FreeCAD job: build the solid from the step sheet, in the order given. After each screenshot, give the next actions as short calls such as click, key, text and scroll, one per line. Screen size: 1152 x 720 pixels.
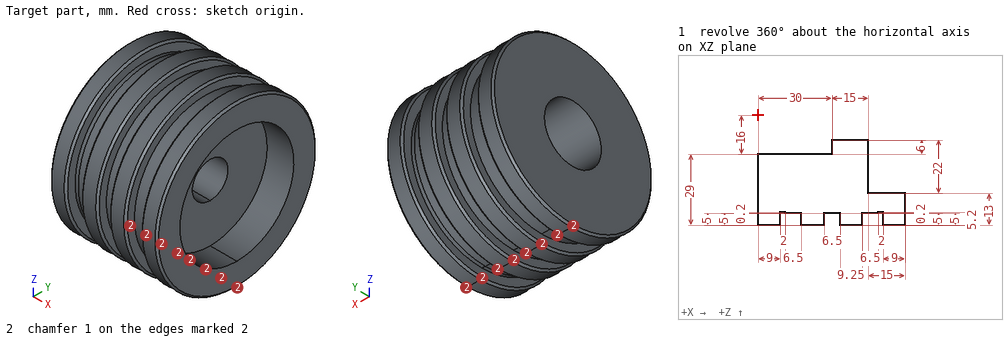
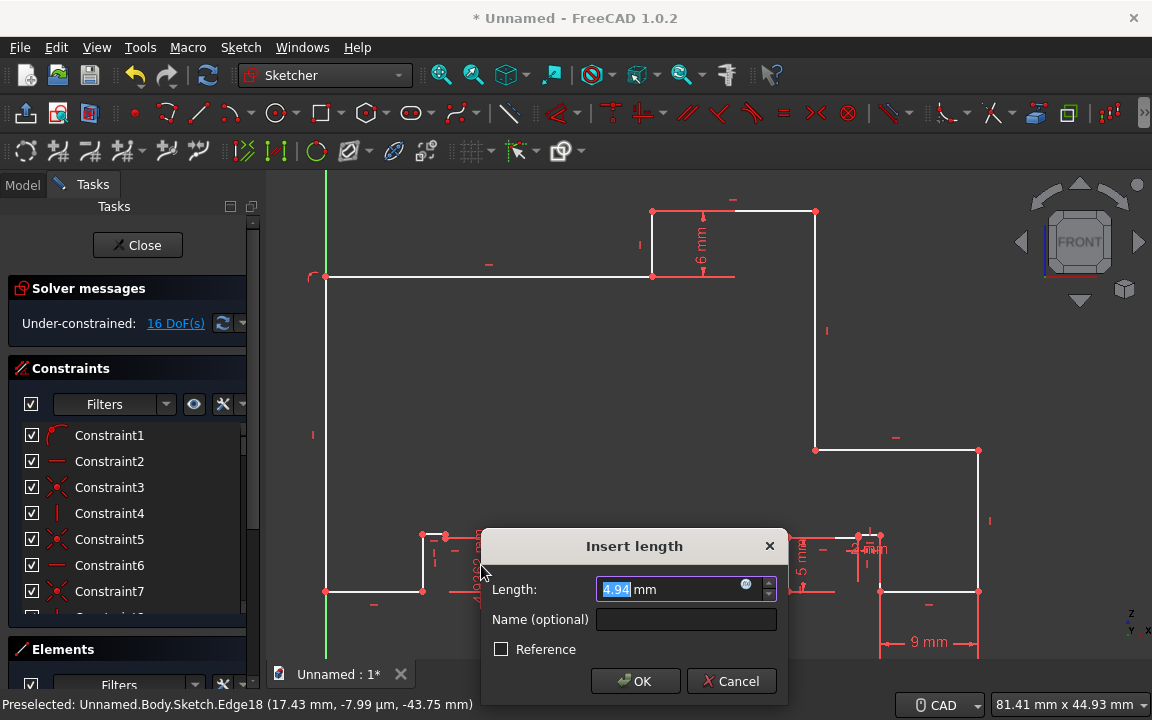
text(5)
key(Return)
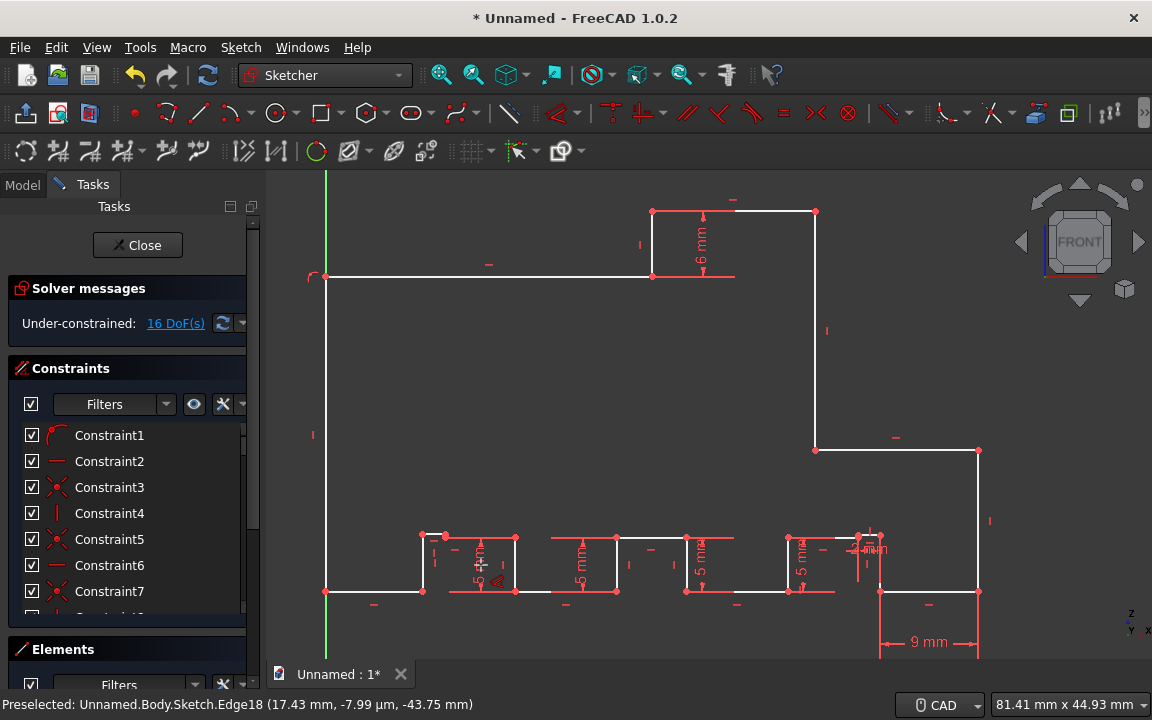
scroll(434, 534, up, 4)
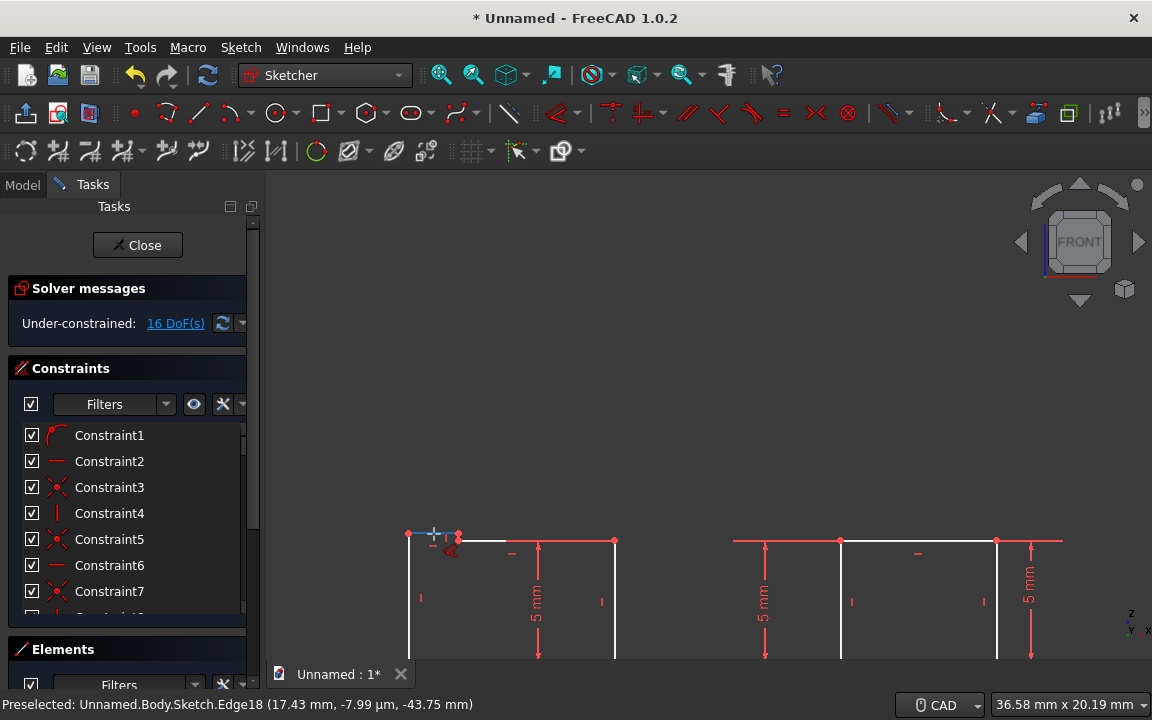
click(434, 533)
click(434, 567)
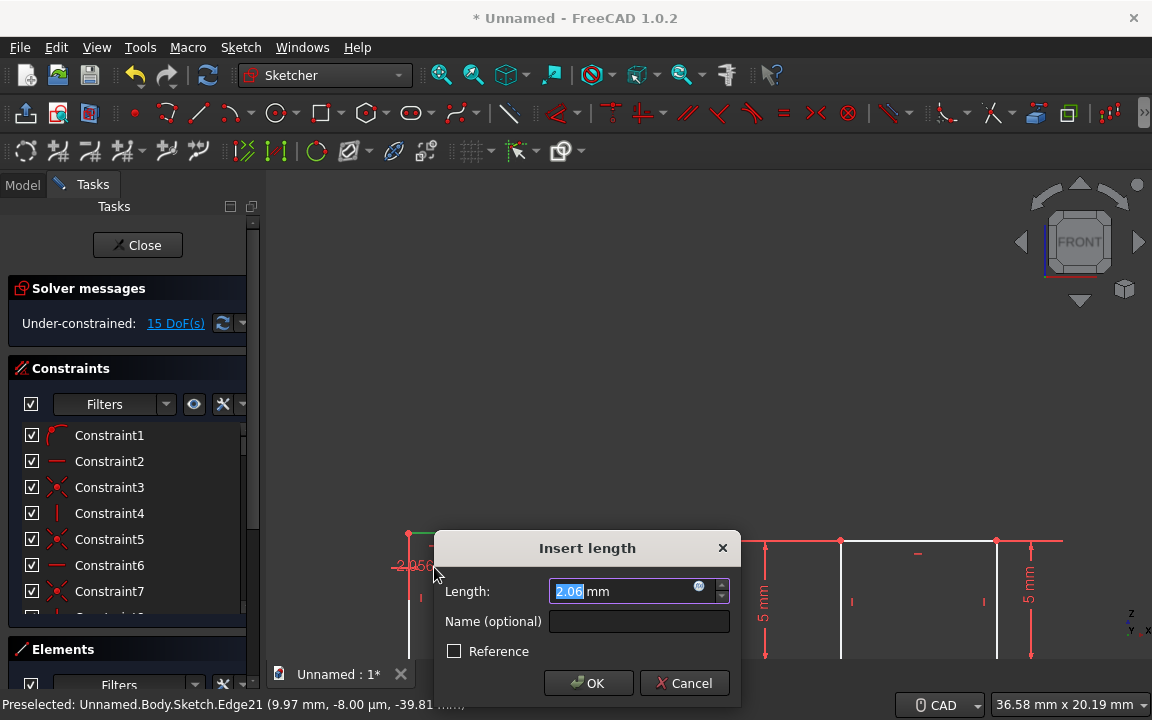
text(2)
key(Return)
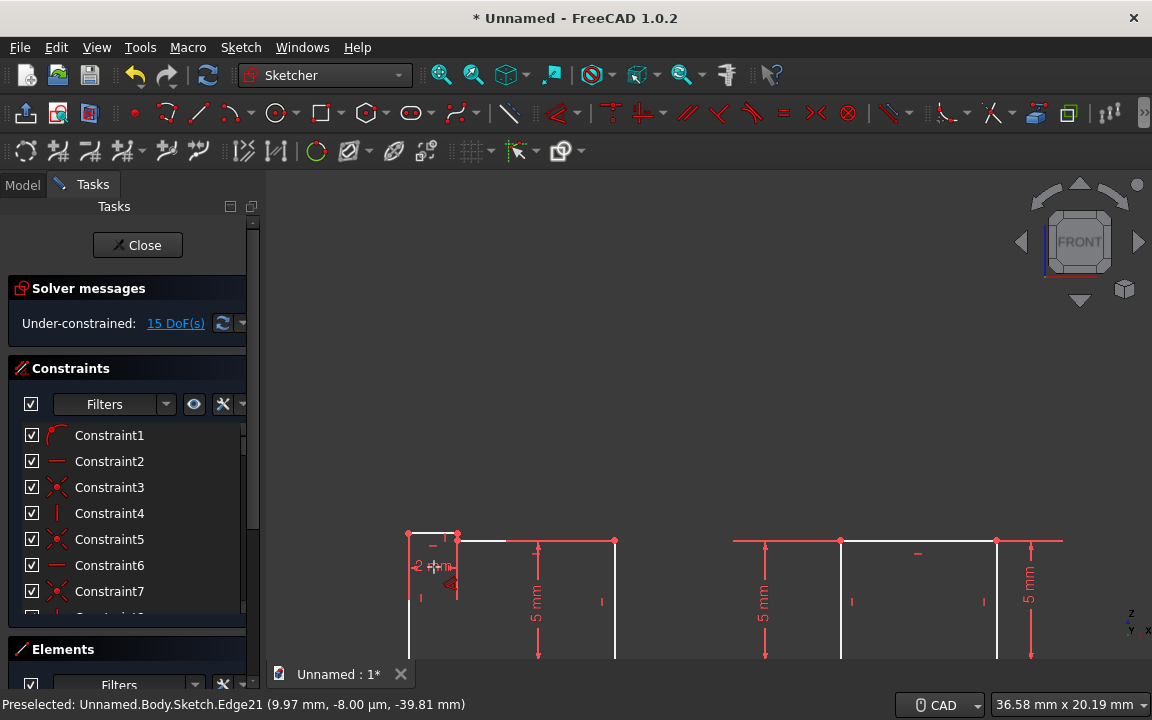
scroll(520, 544, down, 6)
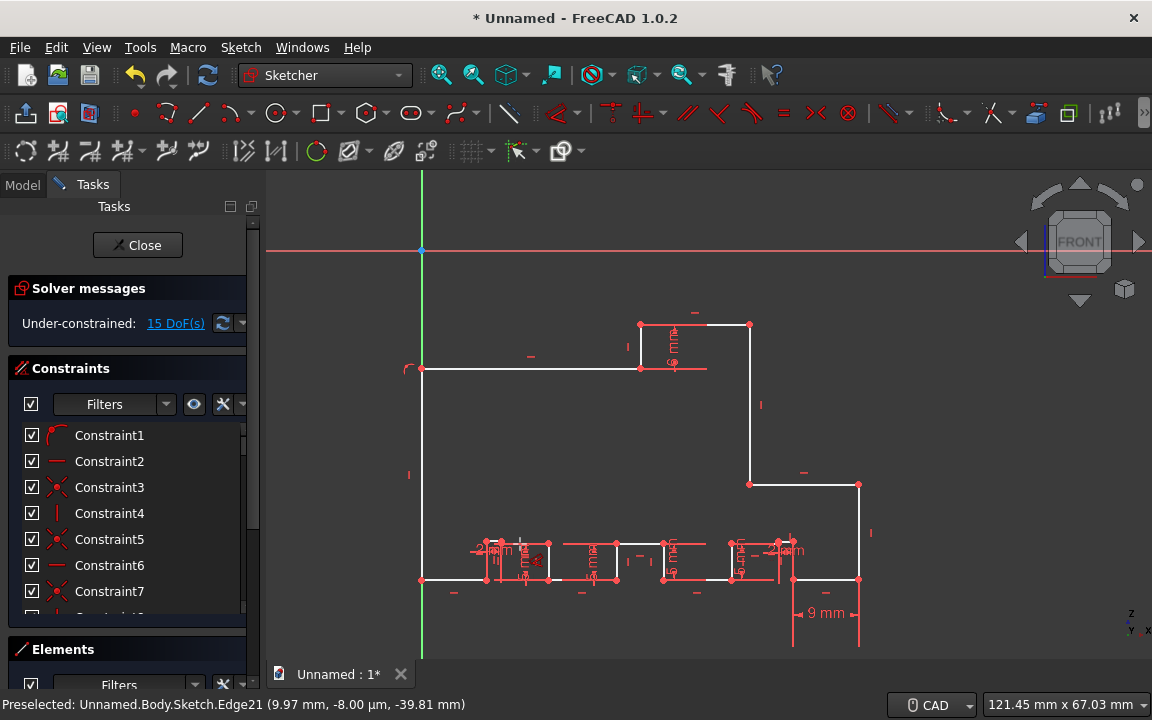
click(467, 580)
click(454, 614)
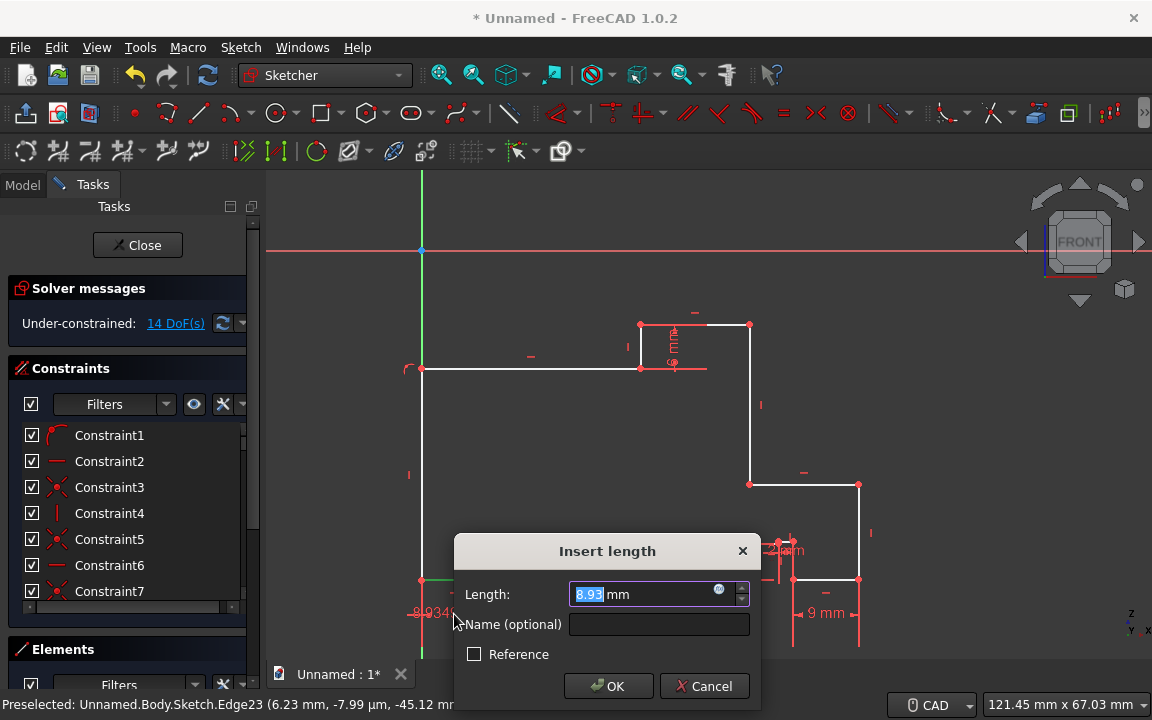
text(9)
key(Return)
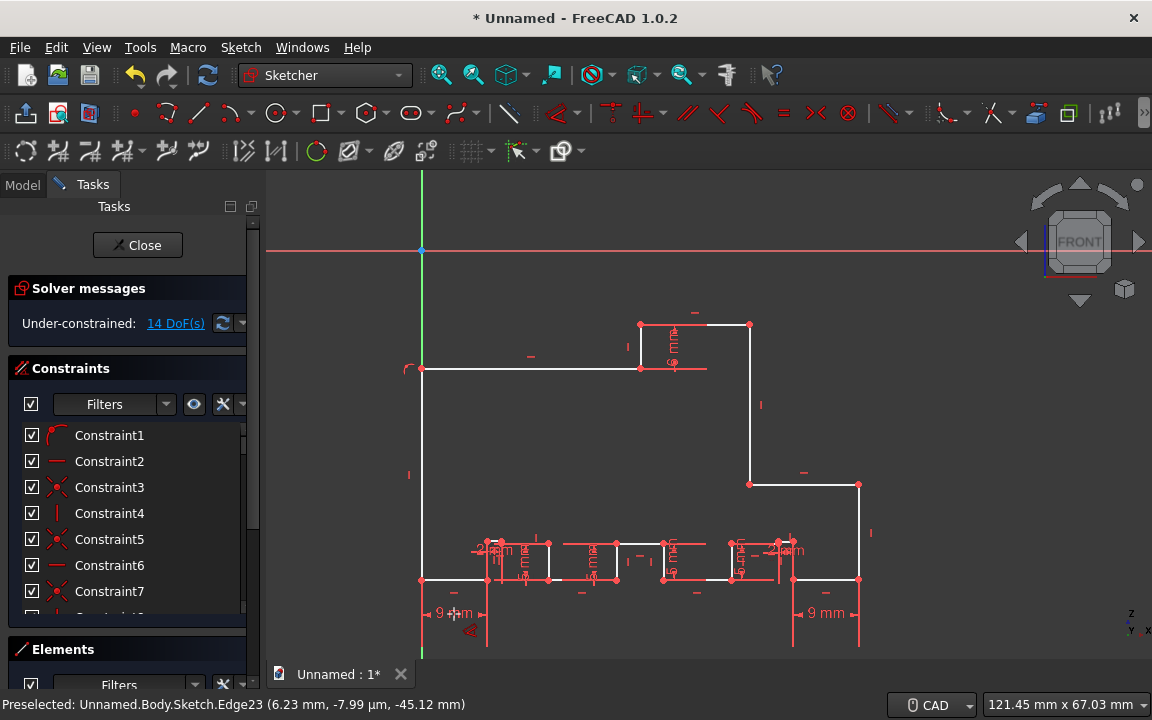
click(487, 369)
click(531, 335)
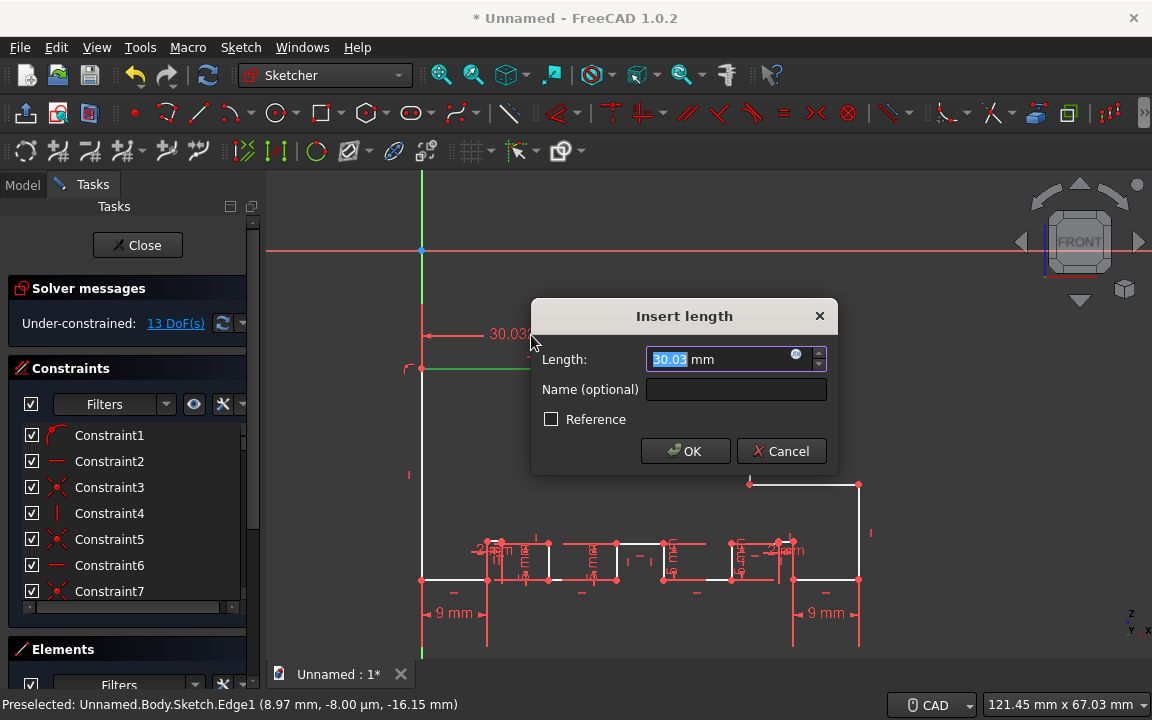
text(30)
key(Return)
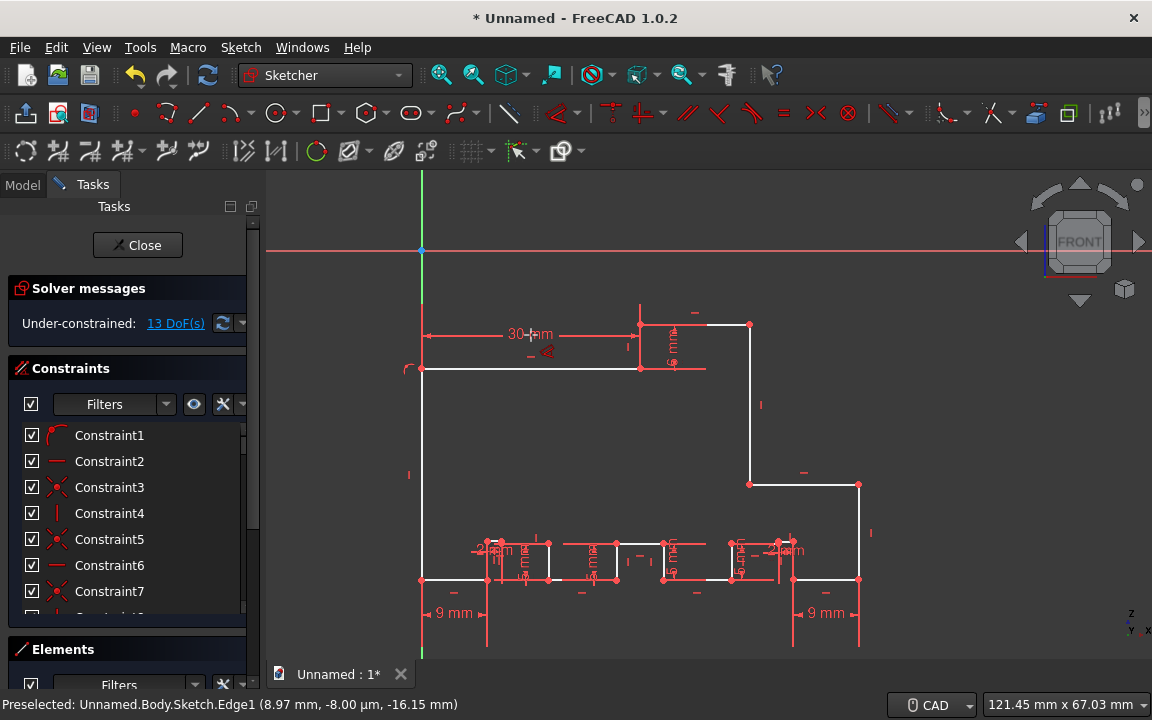
click(673, 325)
click(695, 291)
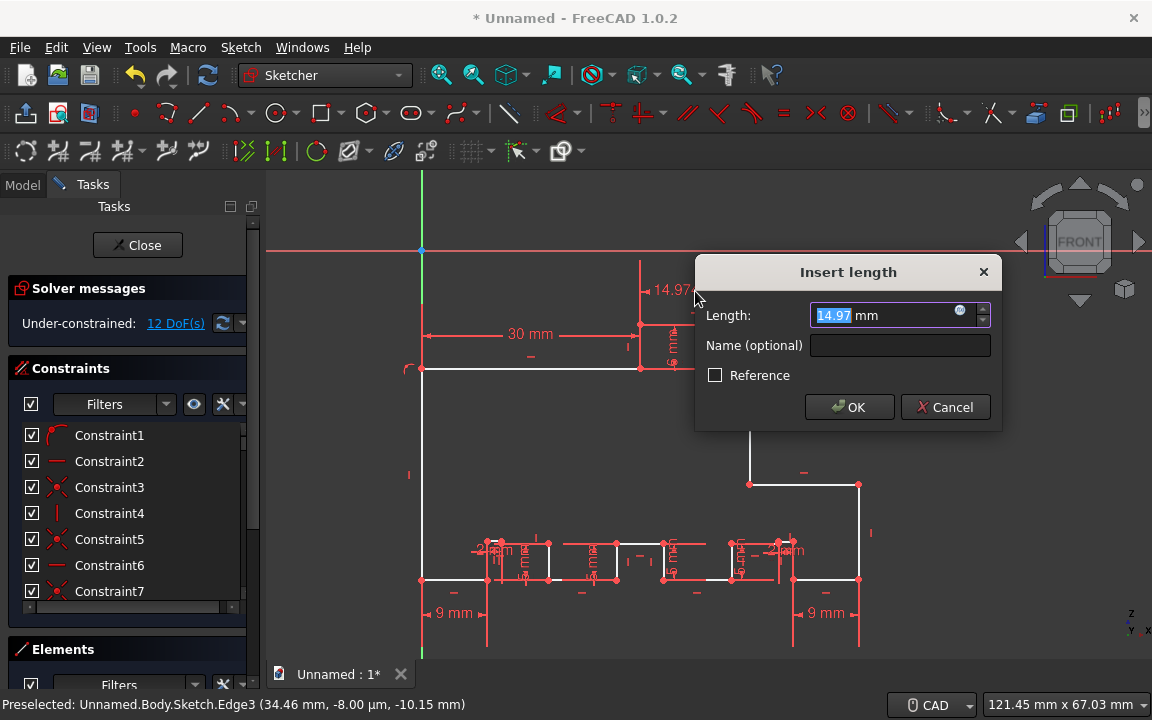
text(15)
key(Return)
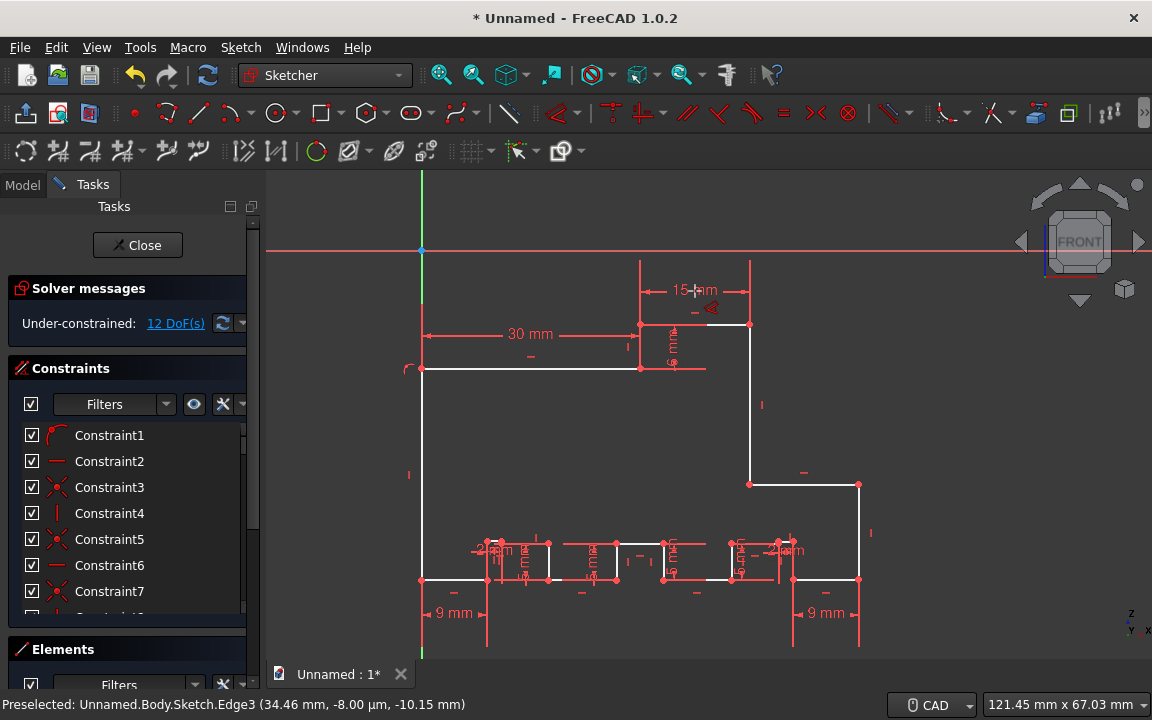
click(750, 373)
click(784, 405)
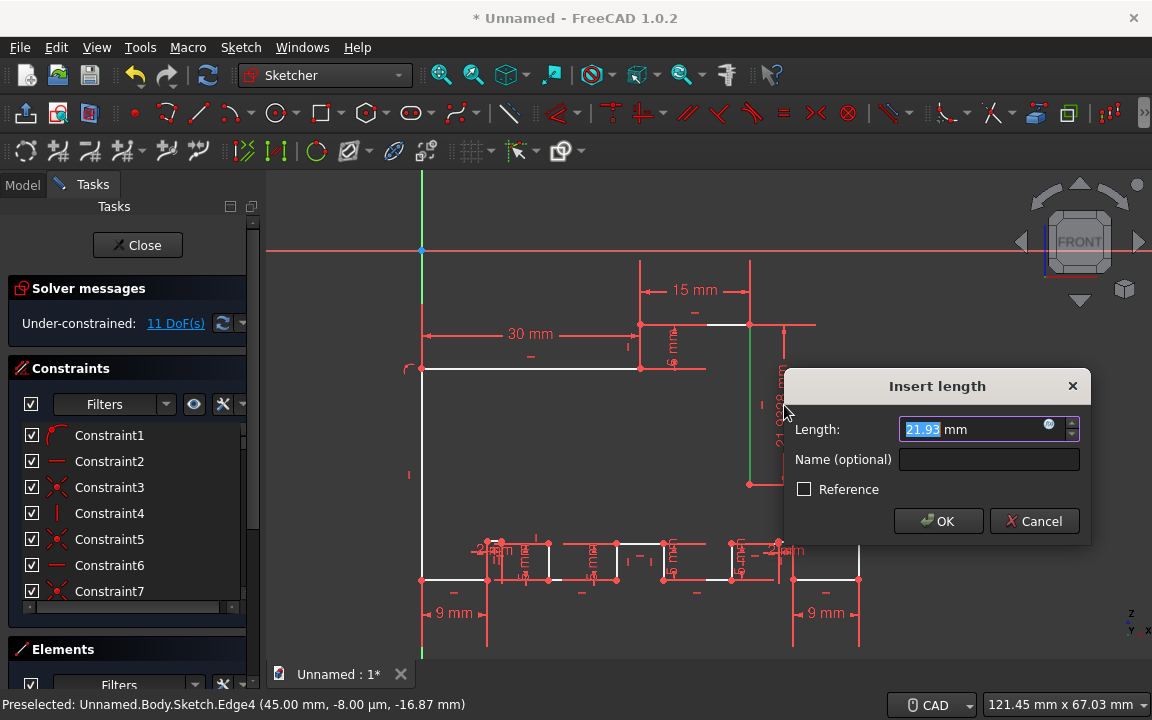
text(22)
key(Return)